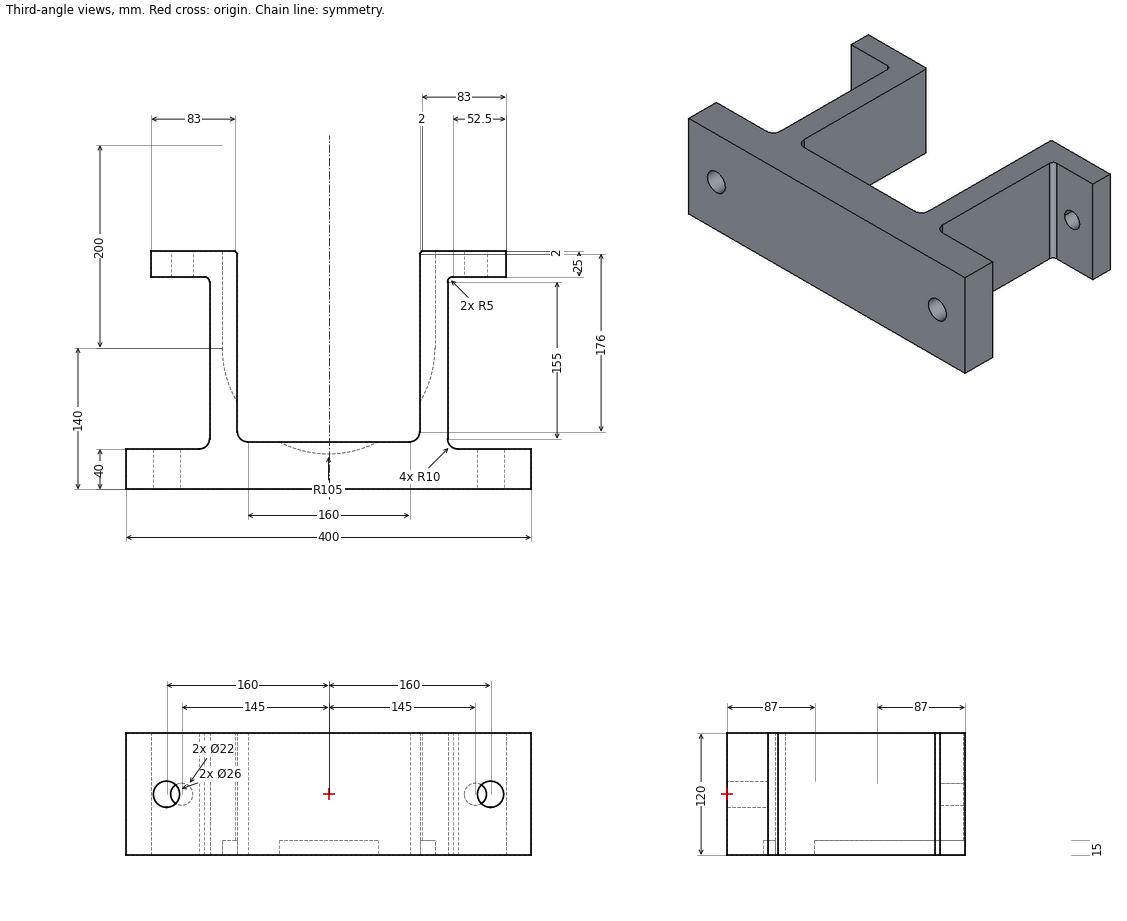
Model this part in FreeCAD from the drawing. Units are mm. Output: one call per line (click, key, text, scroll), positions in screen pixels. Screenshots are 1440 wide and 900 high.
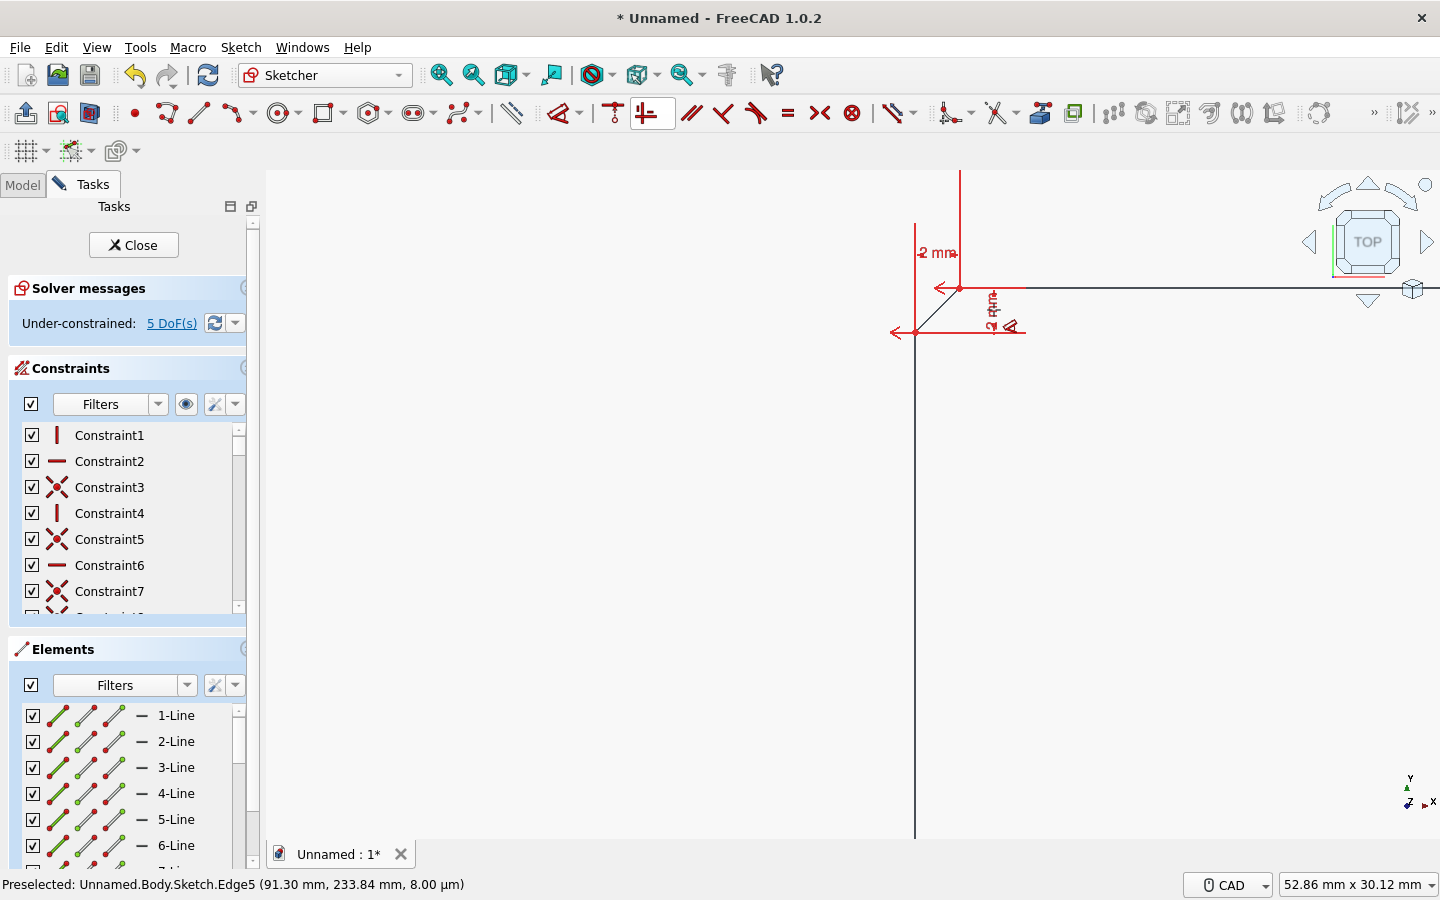
scroll(934, 313, down, 13)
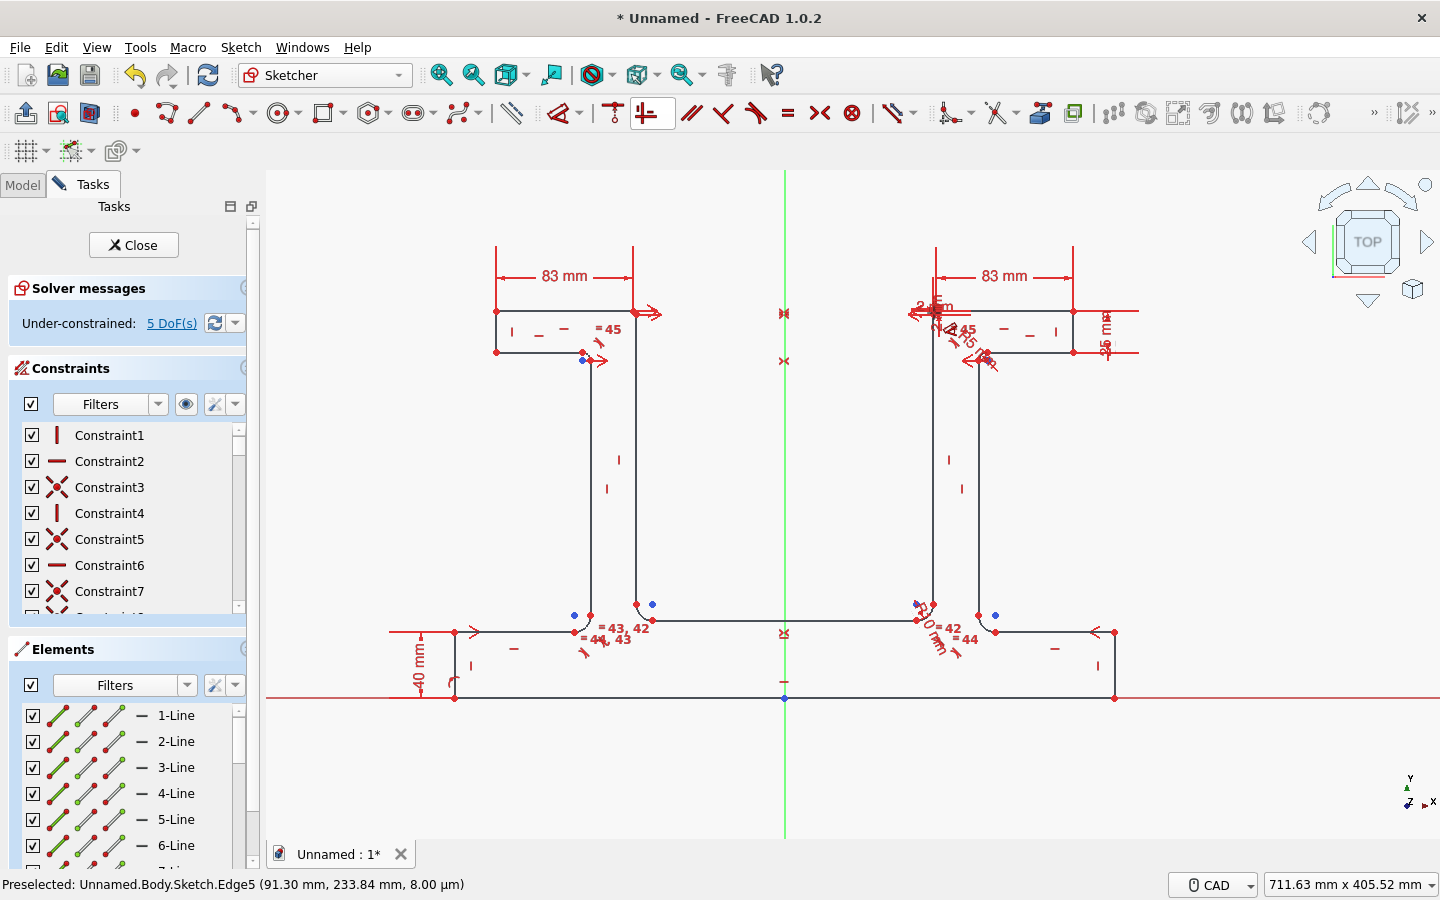
click(979, 539)
click(1013, 488)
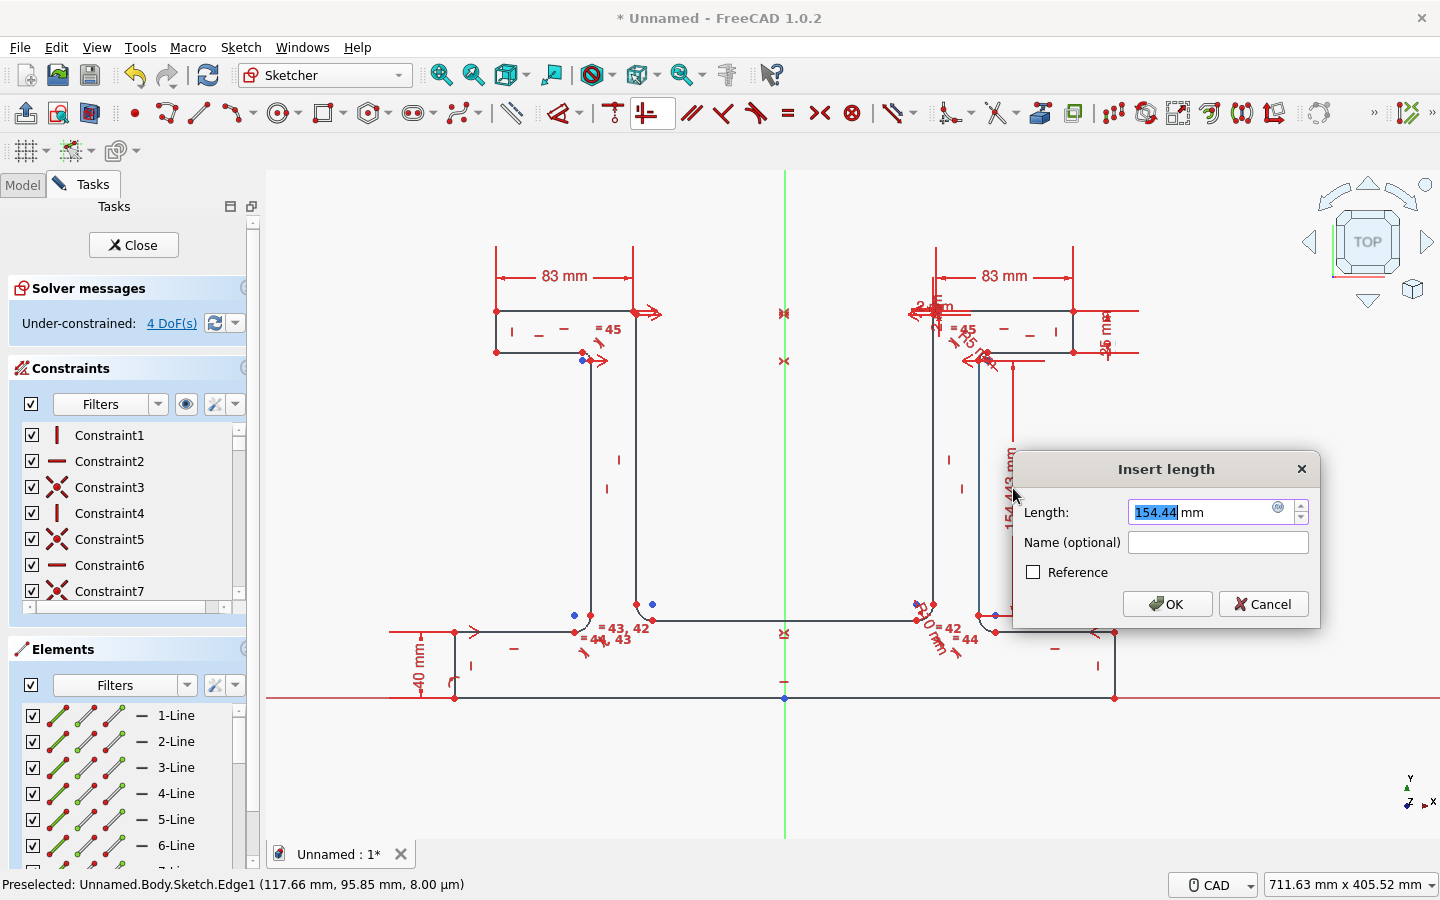
text(155)
key(Return)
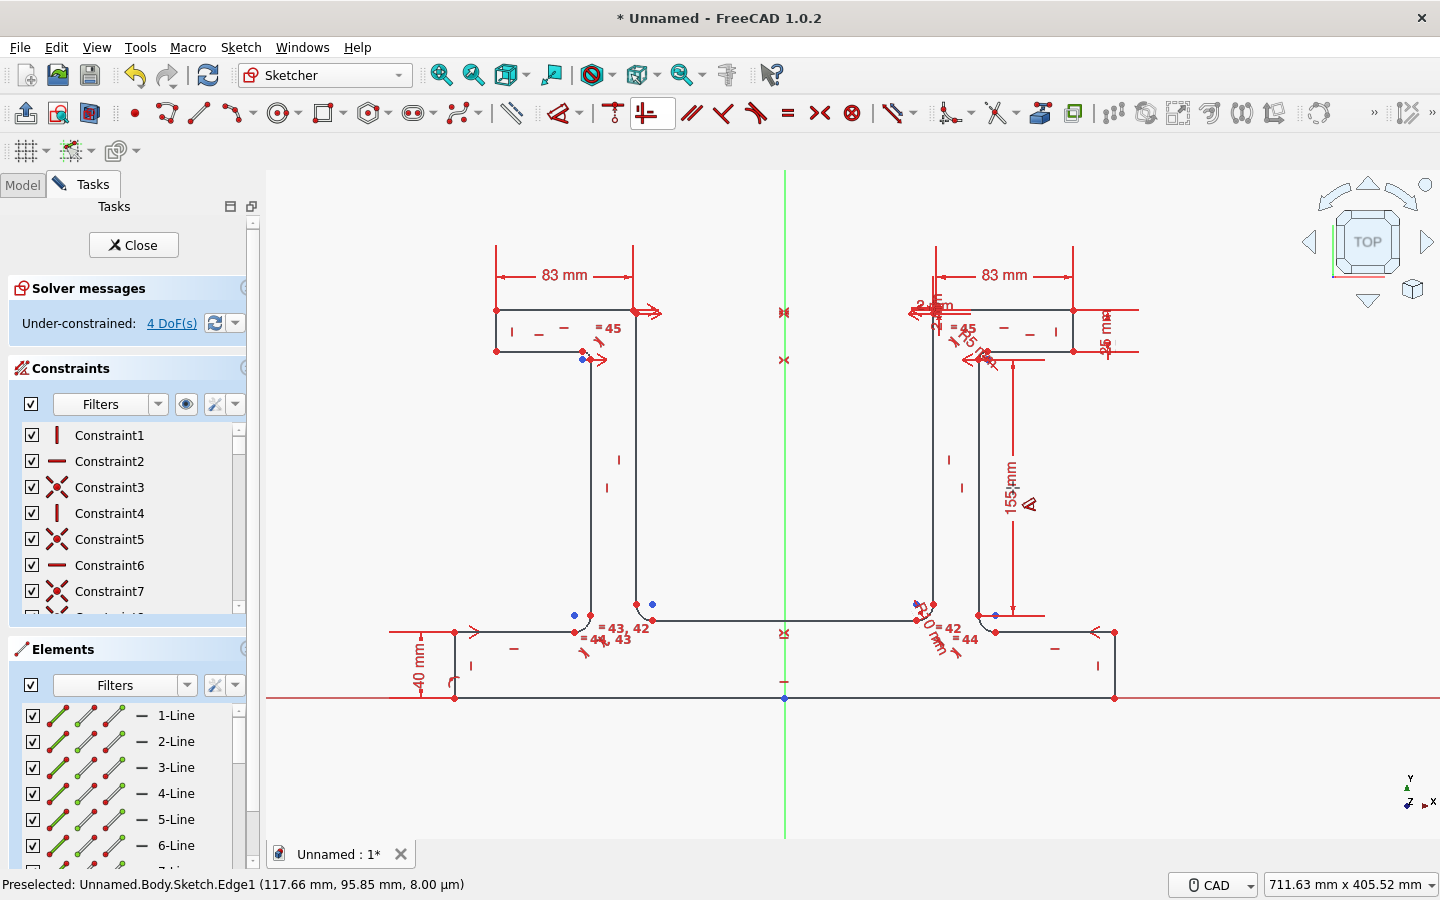
click(933, 401)
click(899, 459)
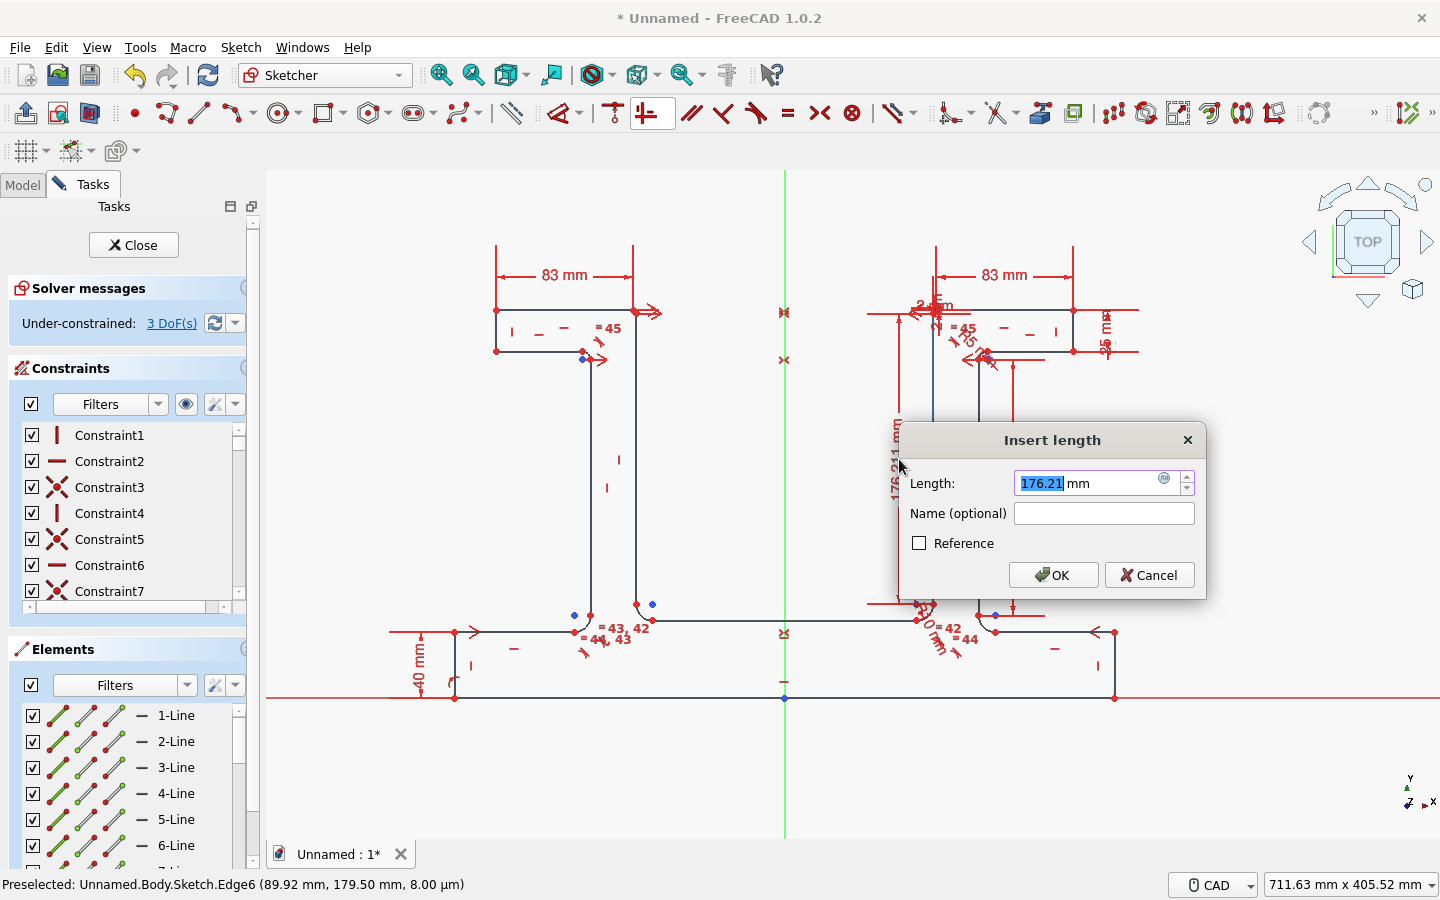
text(176)
key(Return)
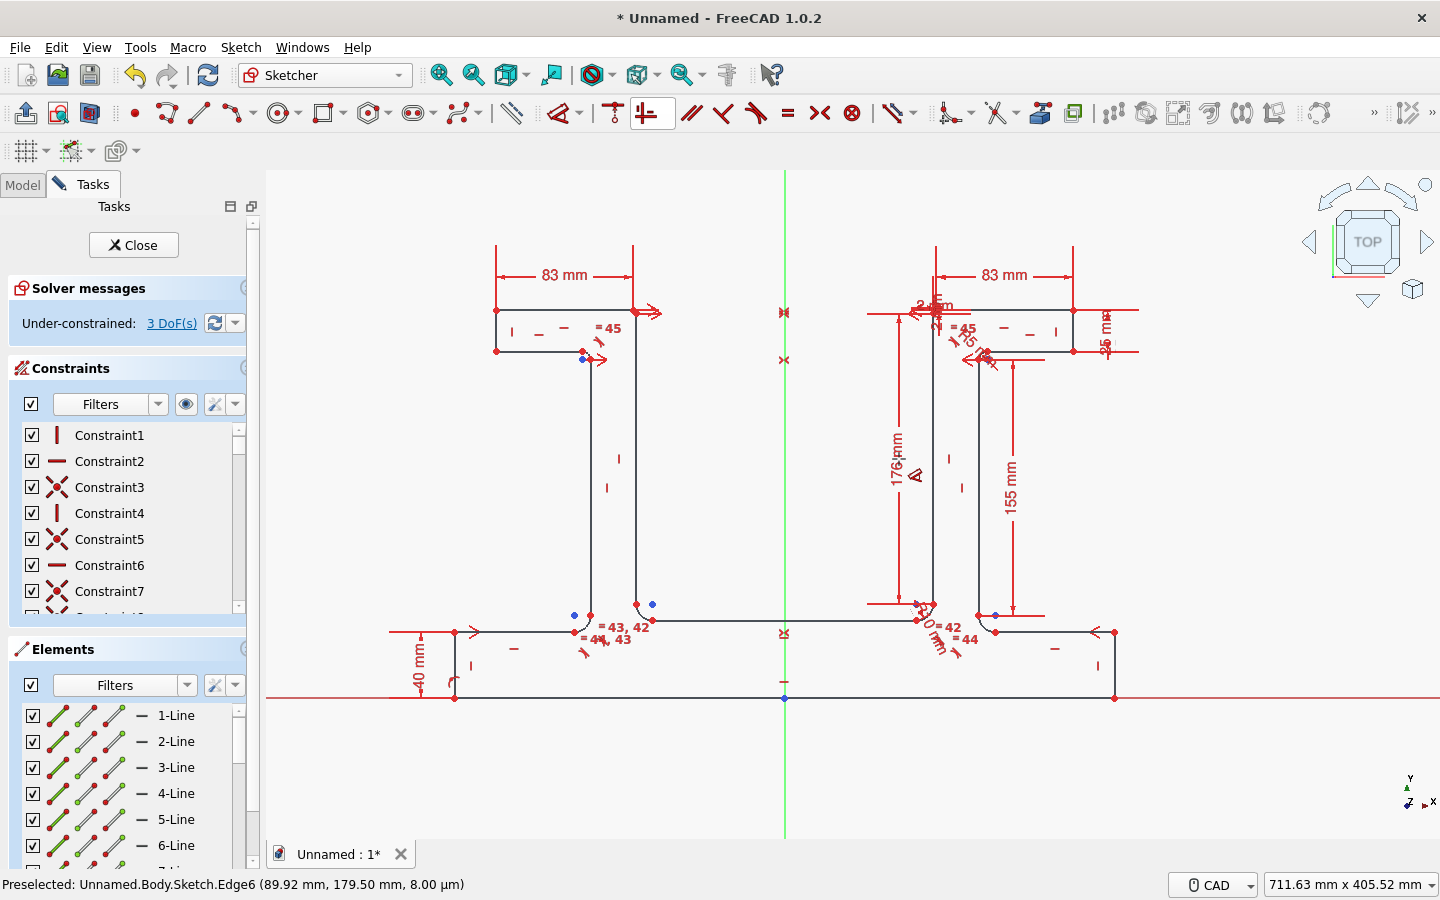
click(838, 621)
click(724, 655)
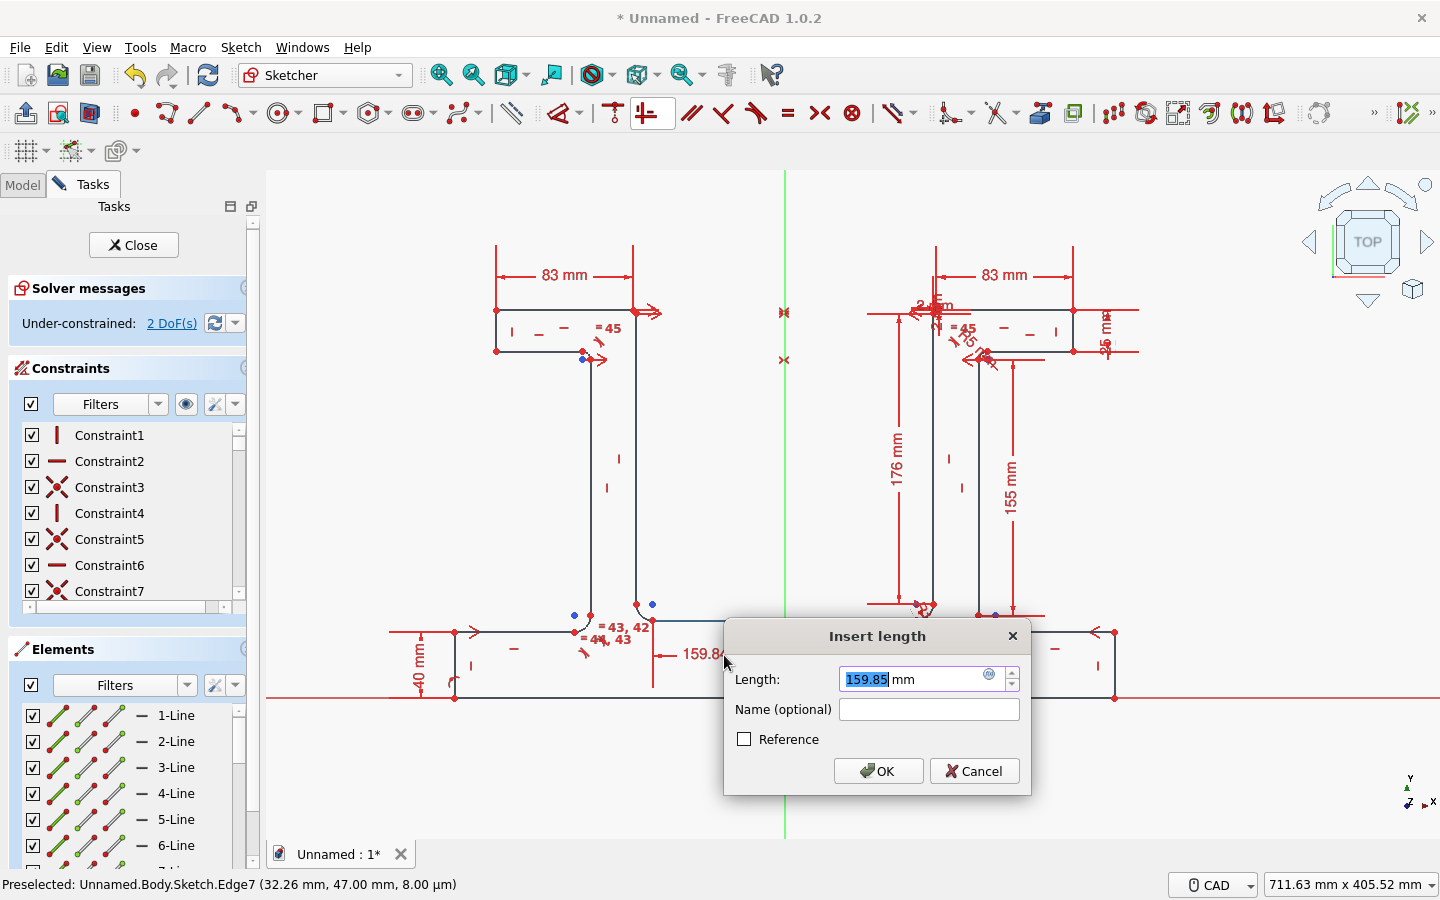
text(160)
key(Return)